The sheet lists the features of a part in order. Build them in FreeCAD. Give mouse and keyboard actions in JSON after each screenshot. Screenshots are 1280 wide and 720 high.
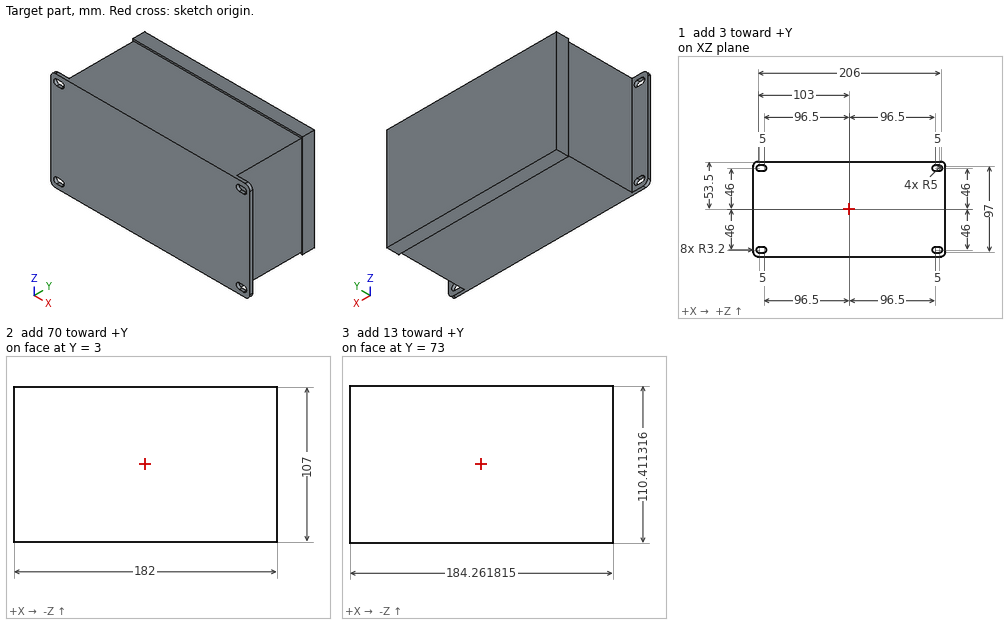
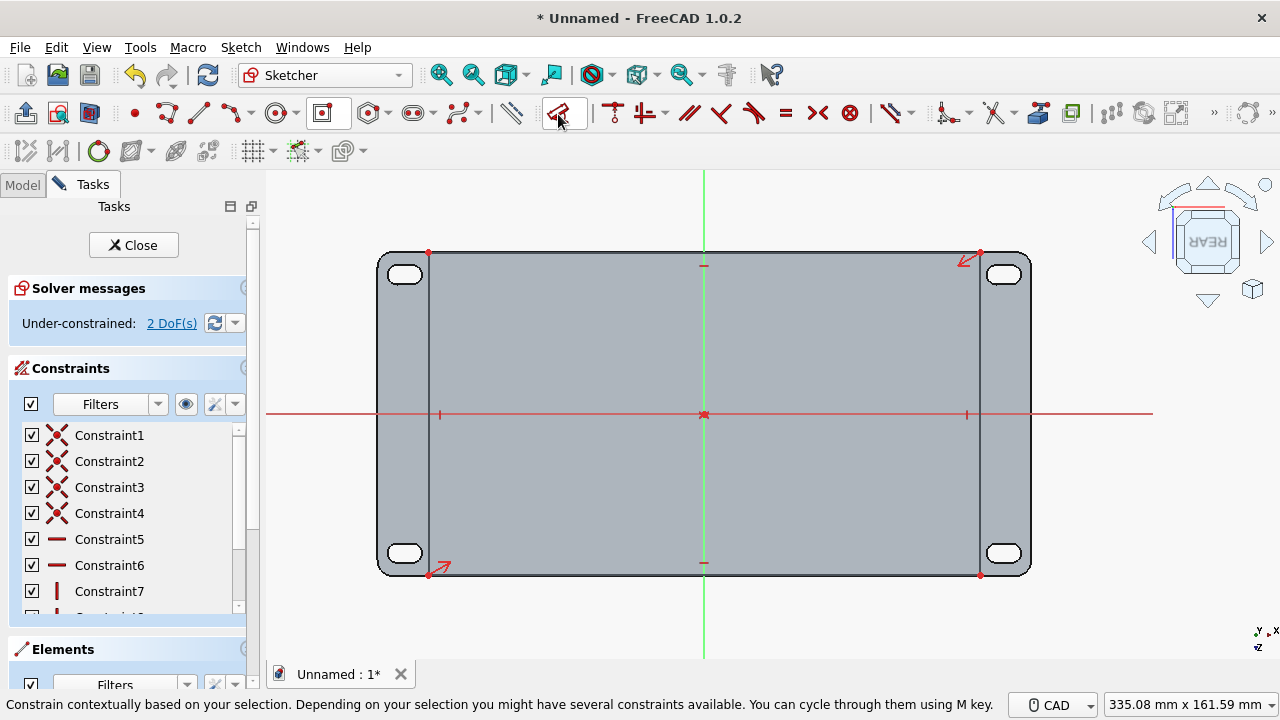
{"action": "left_click", "coordinate": [594, 575]}
{"action": "left_click", "coordinate": [578, 609]}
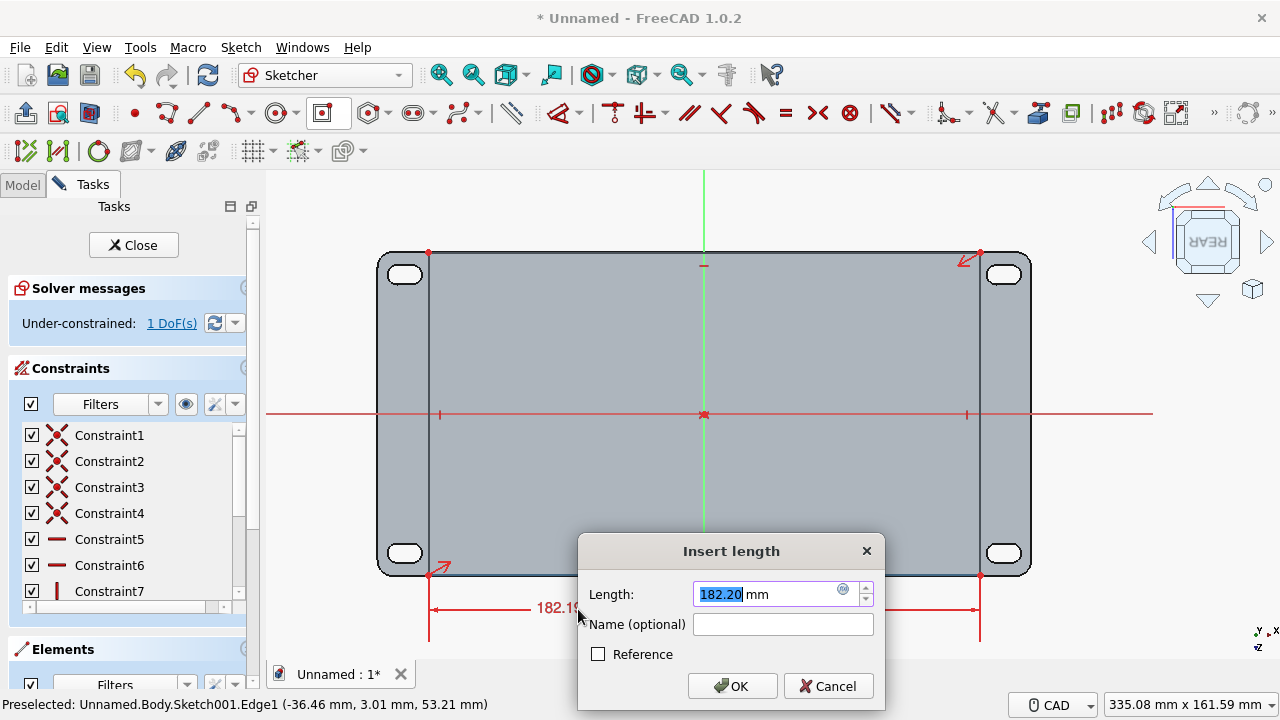
{"action": "type", "text": "182"}
{"action": "key", "text": "Return"}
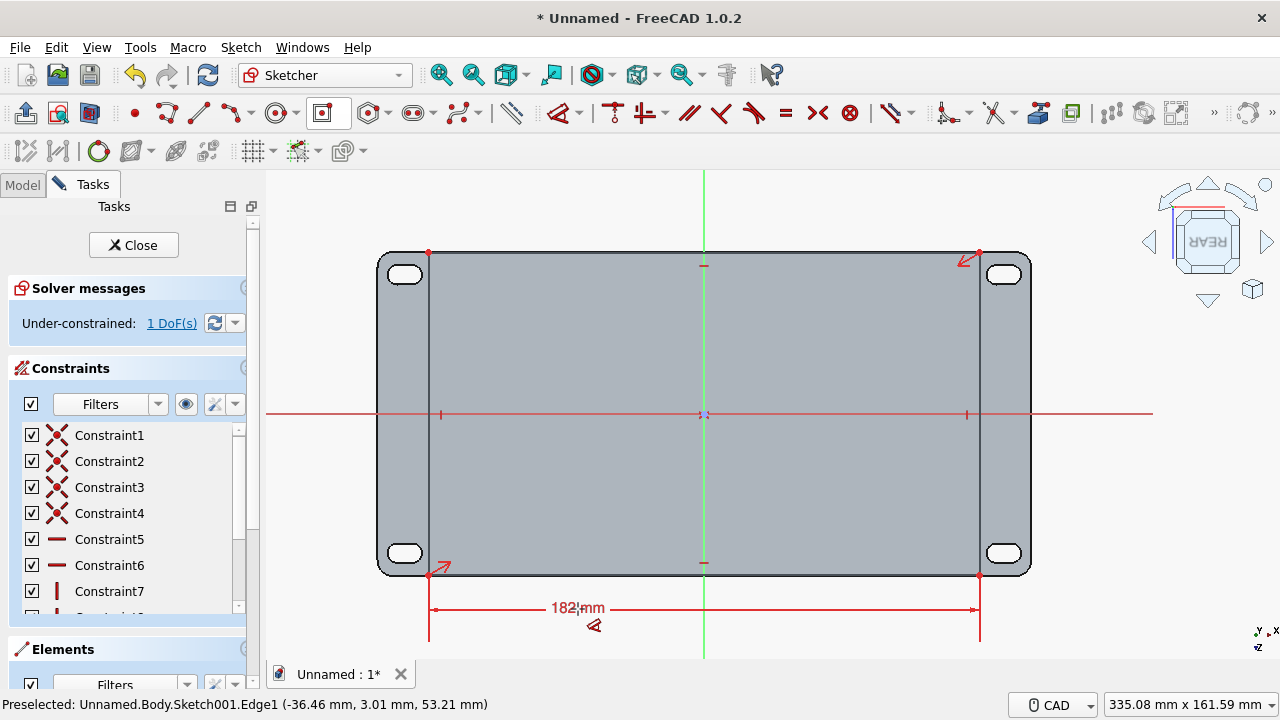
{"action": "left_click", "coordinate": [980, 478]}
{"action": "left_click", "coordinate": [1014, 340]}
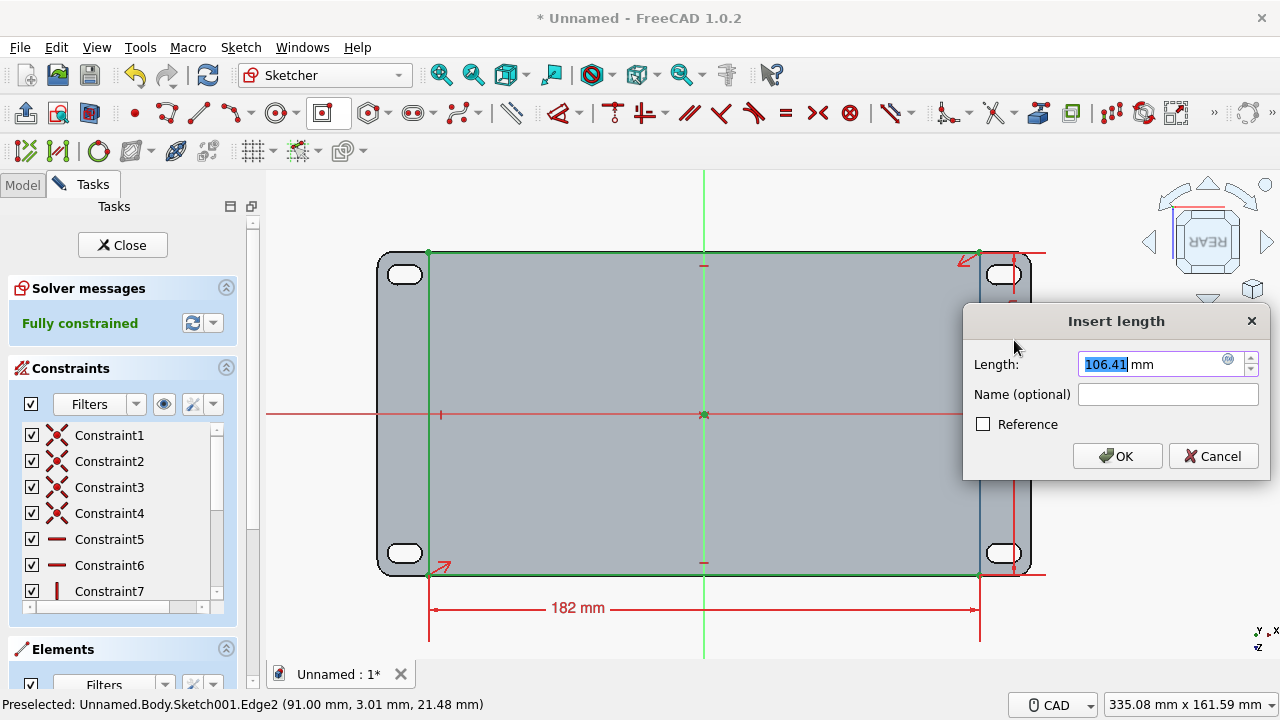
{"action": "type", "text": "107"}
{"action": "key", "text": "Return"}
{"action": "key", "text": "Escape"}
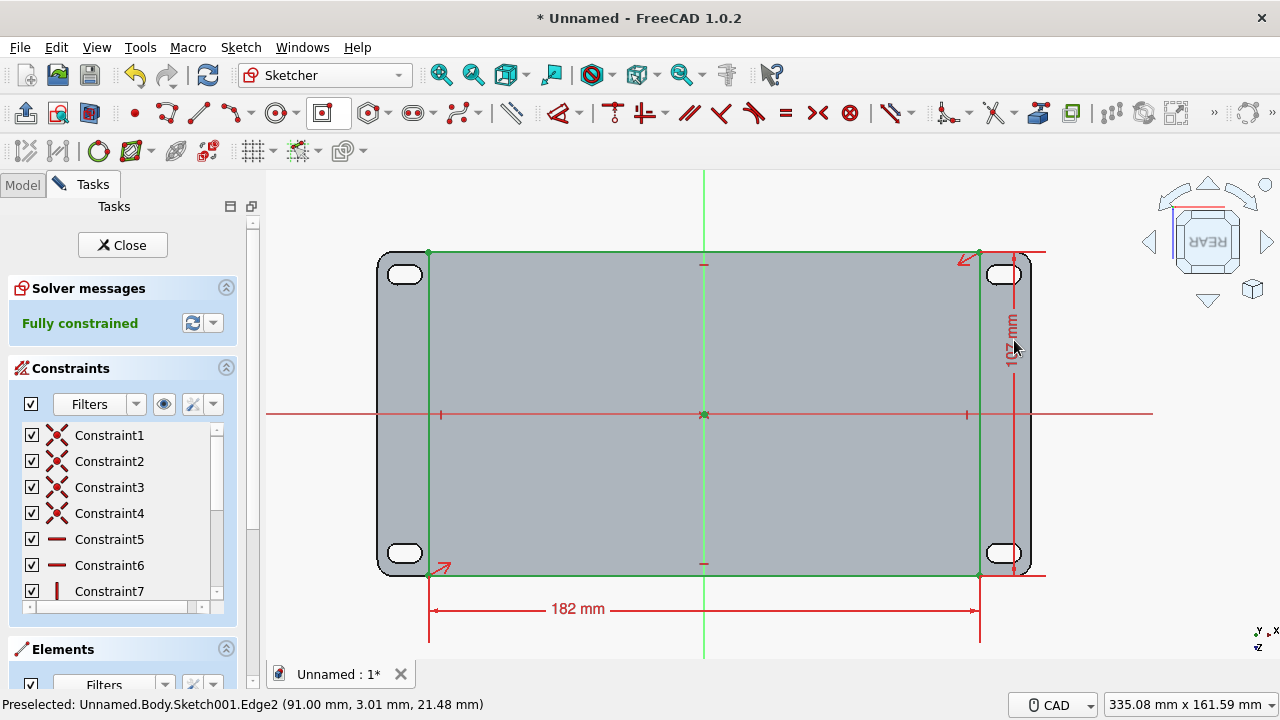
{"action": "left_click", "coordinate": [123, 245]}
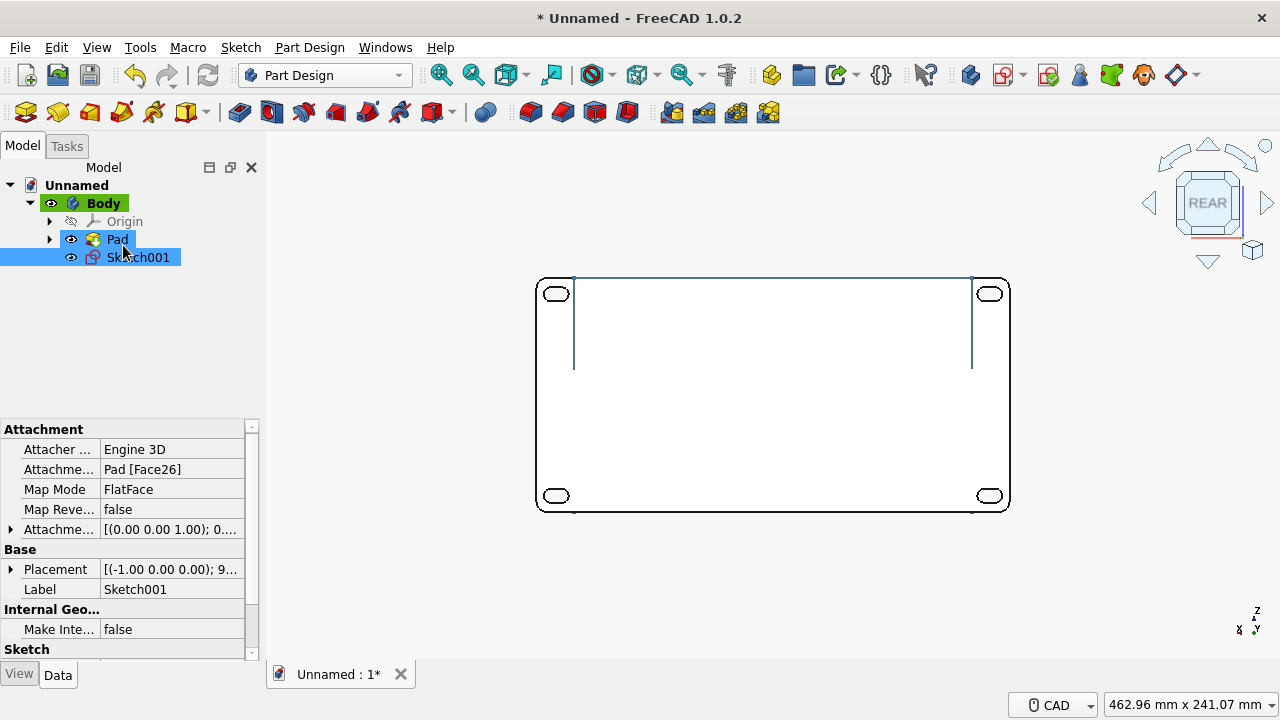
{"action": "left_click", "coordinate": [26, 112]}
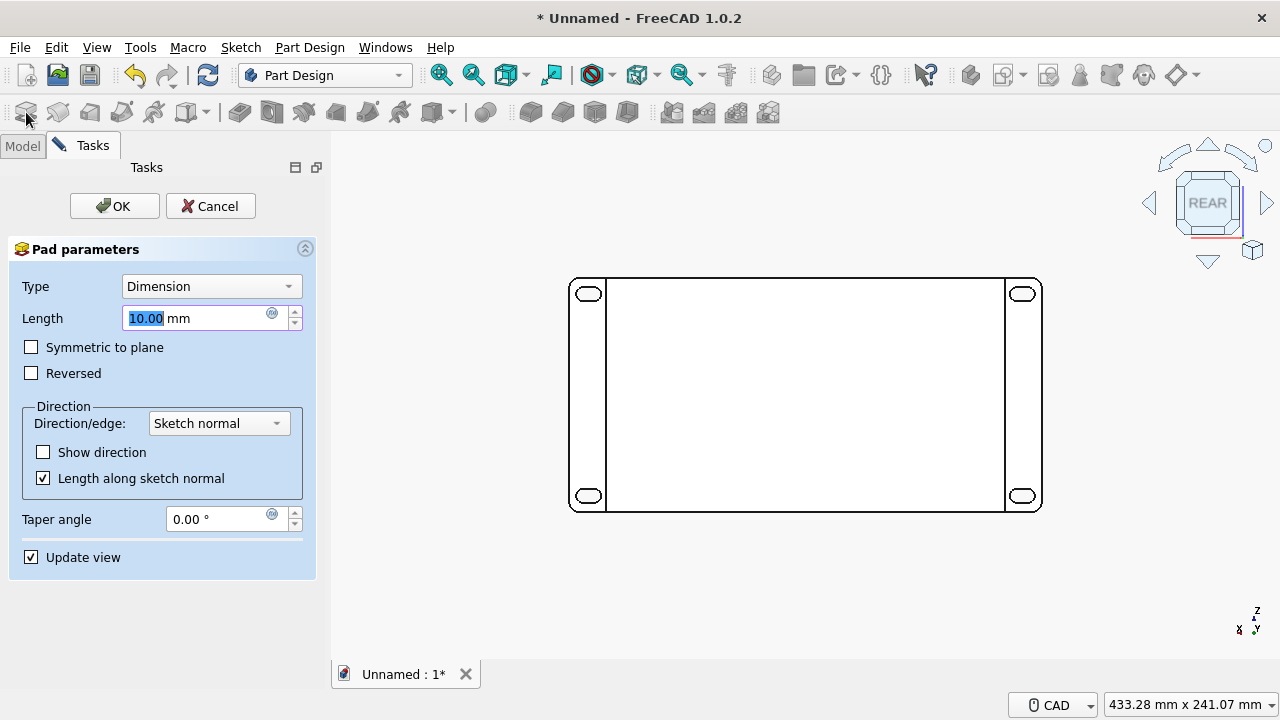
{"action": "type", "text": "70"}
{"action": "key", "text": "Tab"}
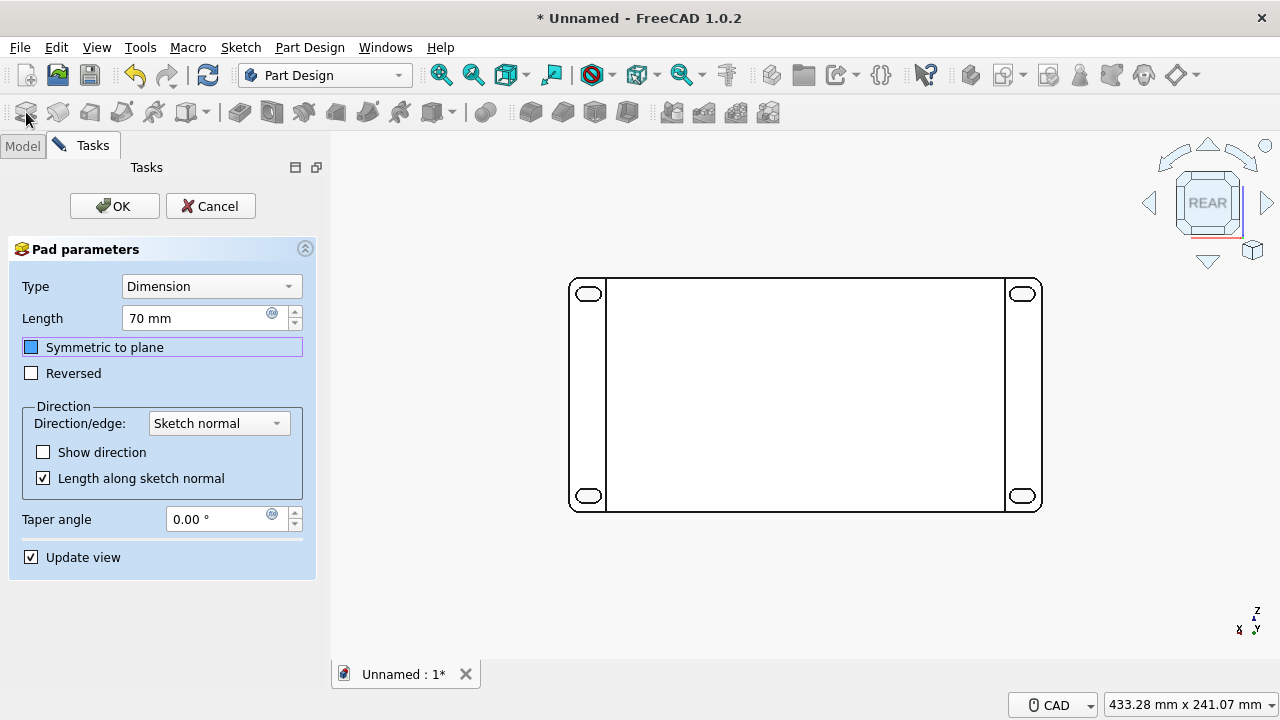
{"action": "left_click", "coordinate": [115, 206]}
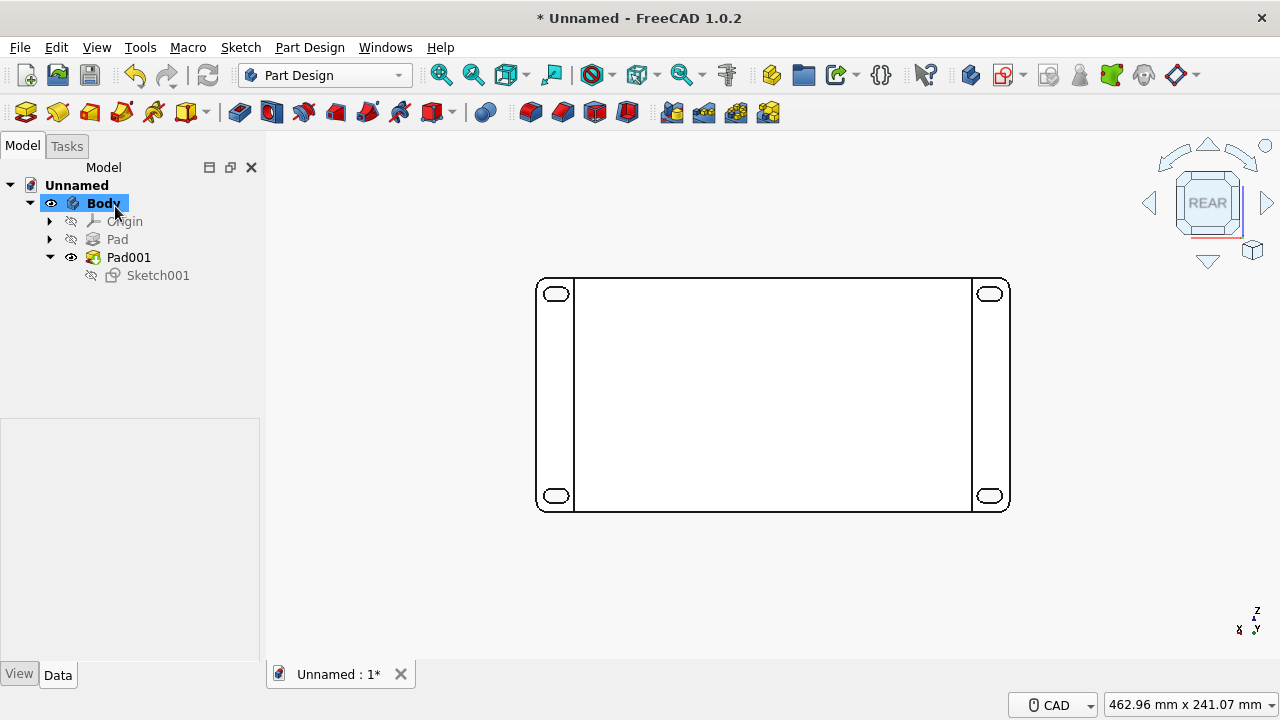
{"action": "left_click", "coordinate": [716, 394]}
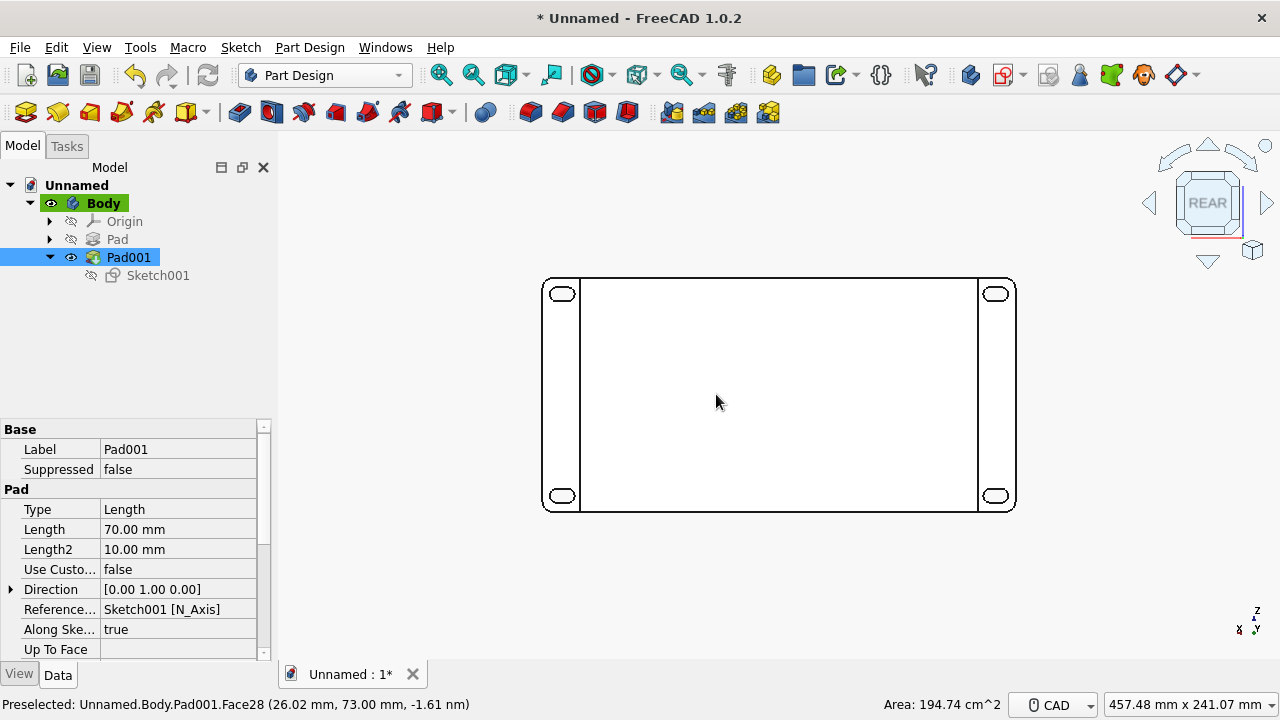
{"action": "left_click", "coordinate": [1004, 76]}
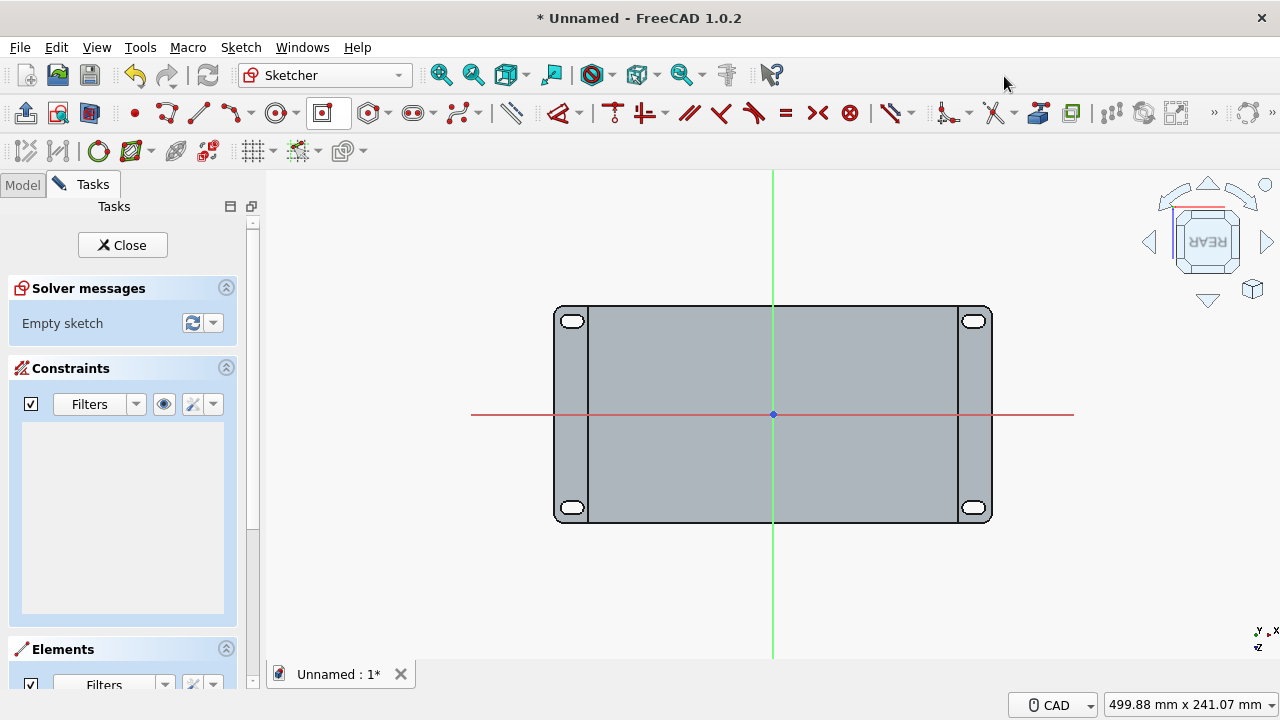
{"action": "scroll", "coordinate": [912, 414], "scroll_direction": "up", "scroll_amount": 2}